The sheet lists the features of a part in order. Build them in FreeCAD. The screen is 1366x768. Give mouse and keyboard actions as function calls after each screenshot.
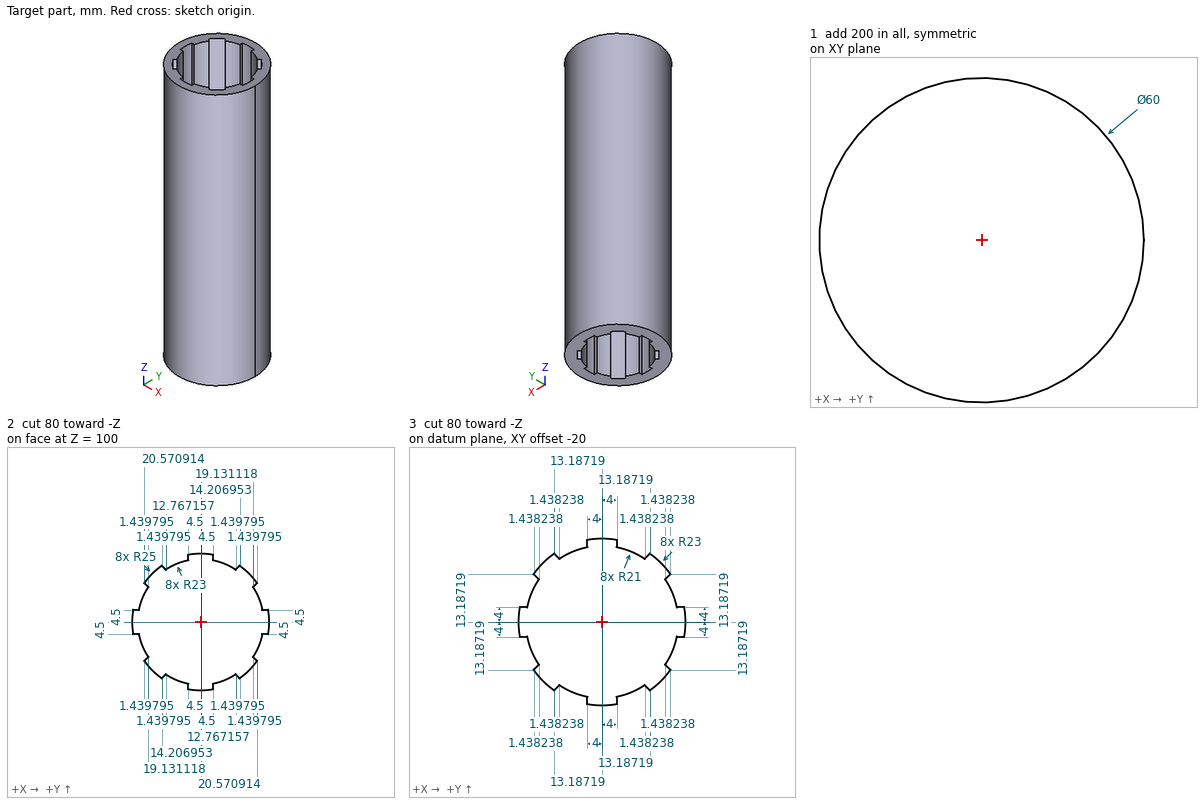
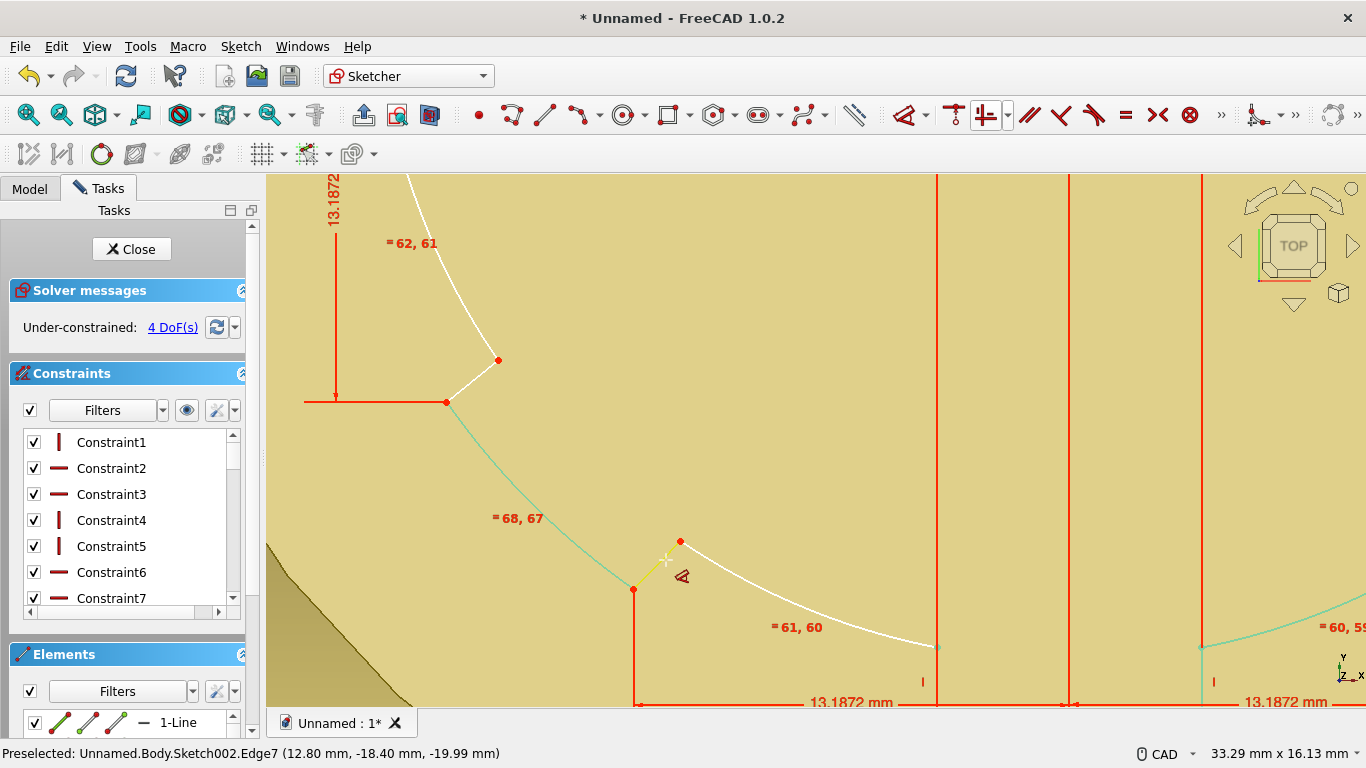
click(667, 556)
click(657, 623)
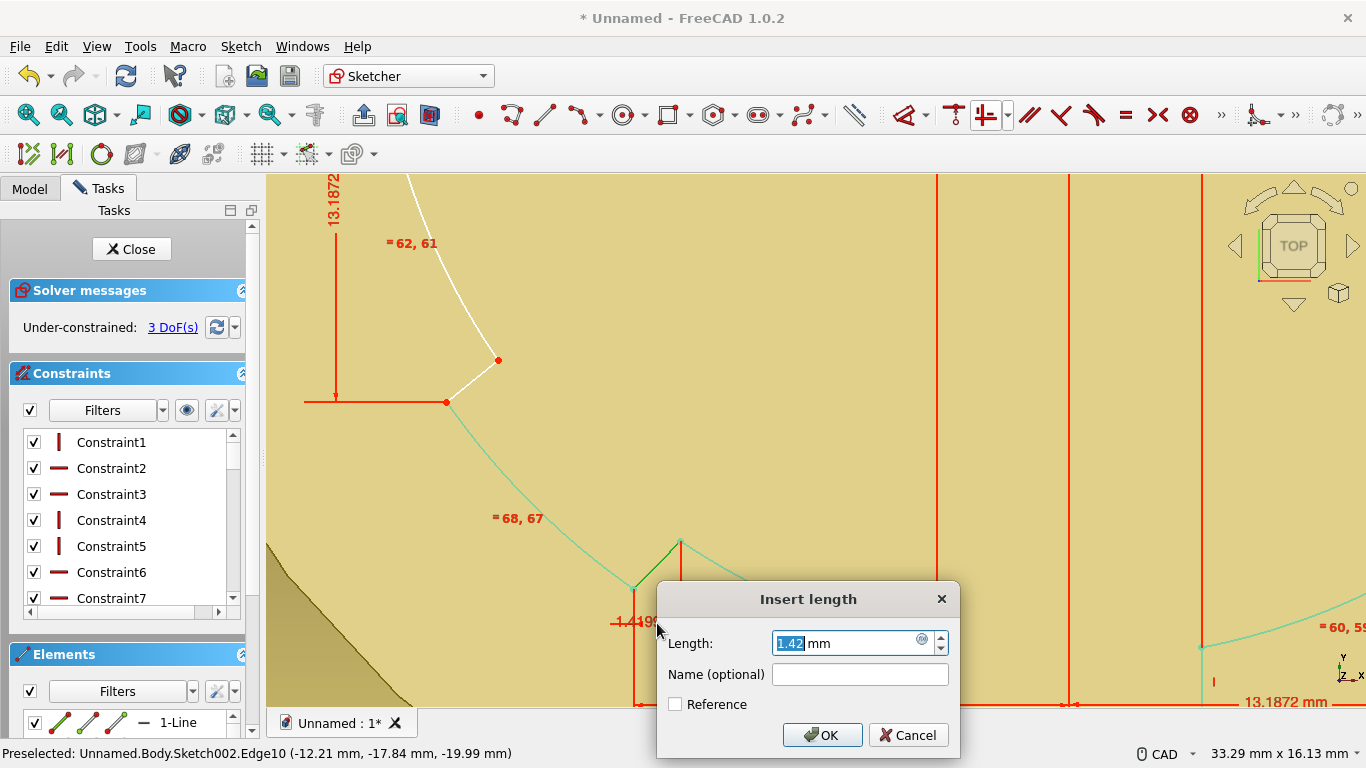
text(1.438238)
key(Return)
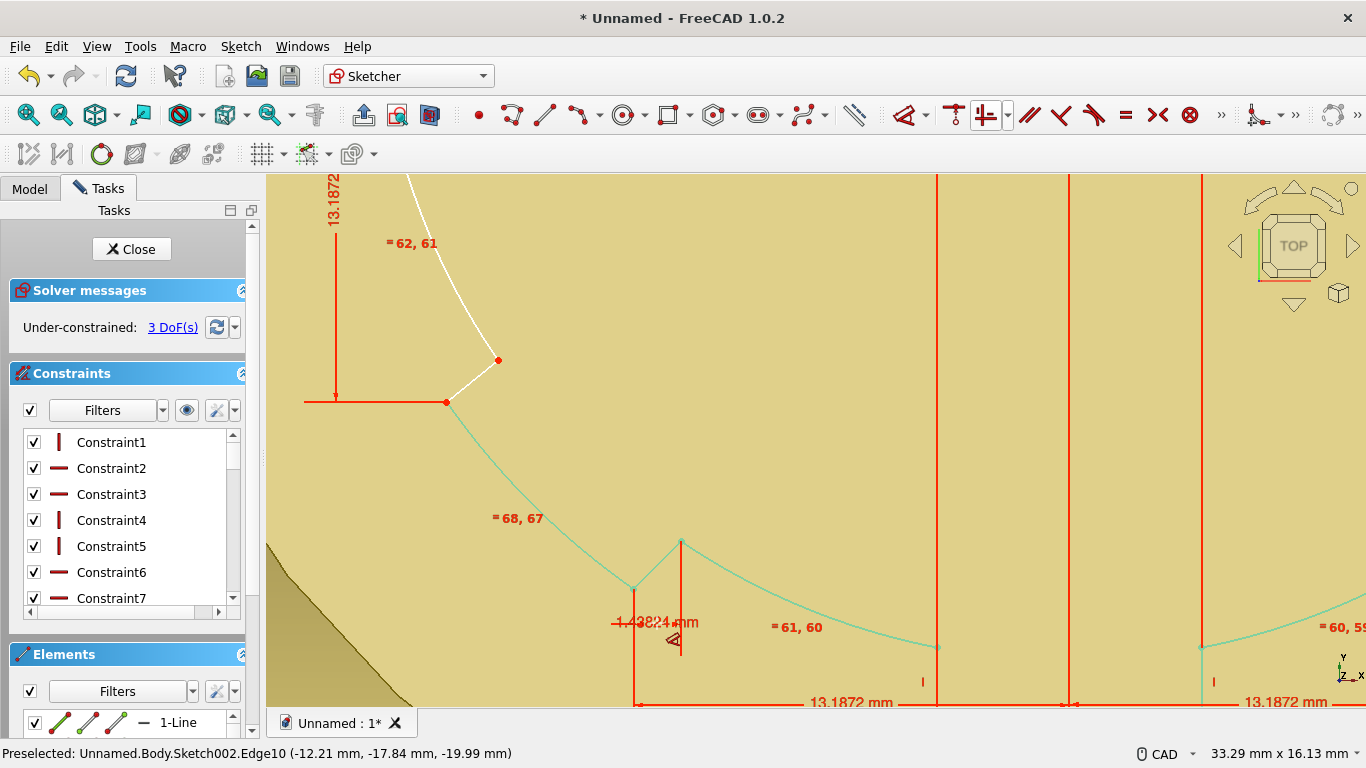
click(462, 390)
click(455, 436)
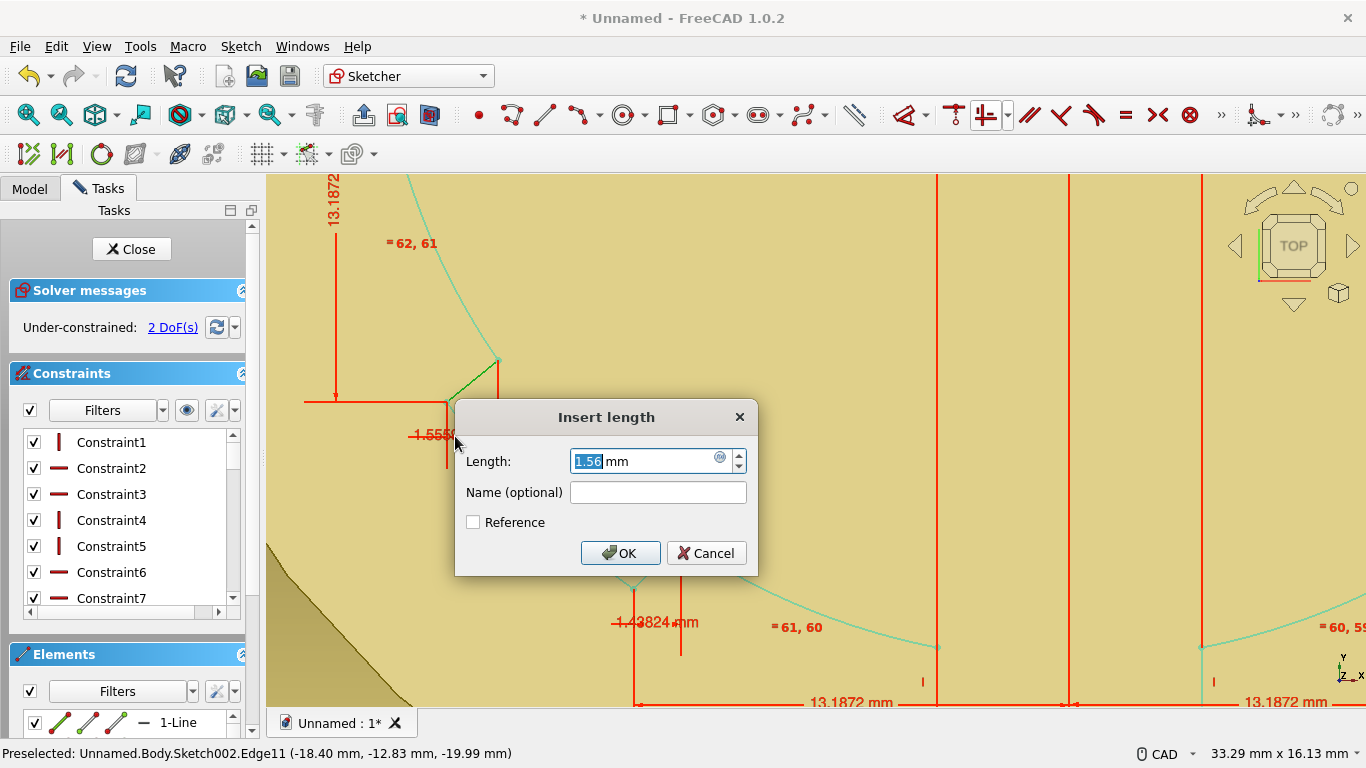
text(1.438238)
key(Return)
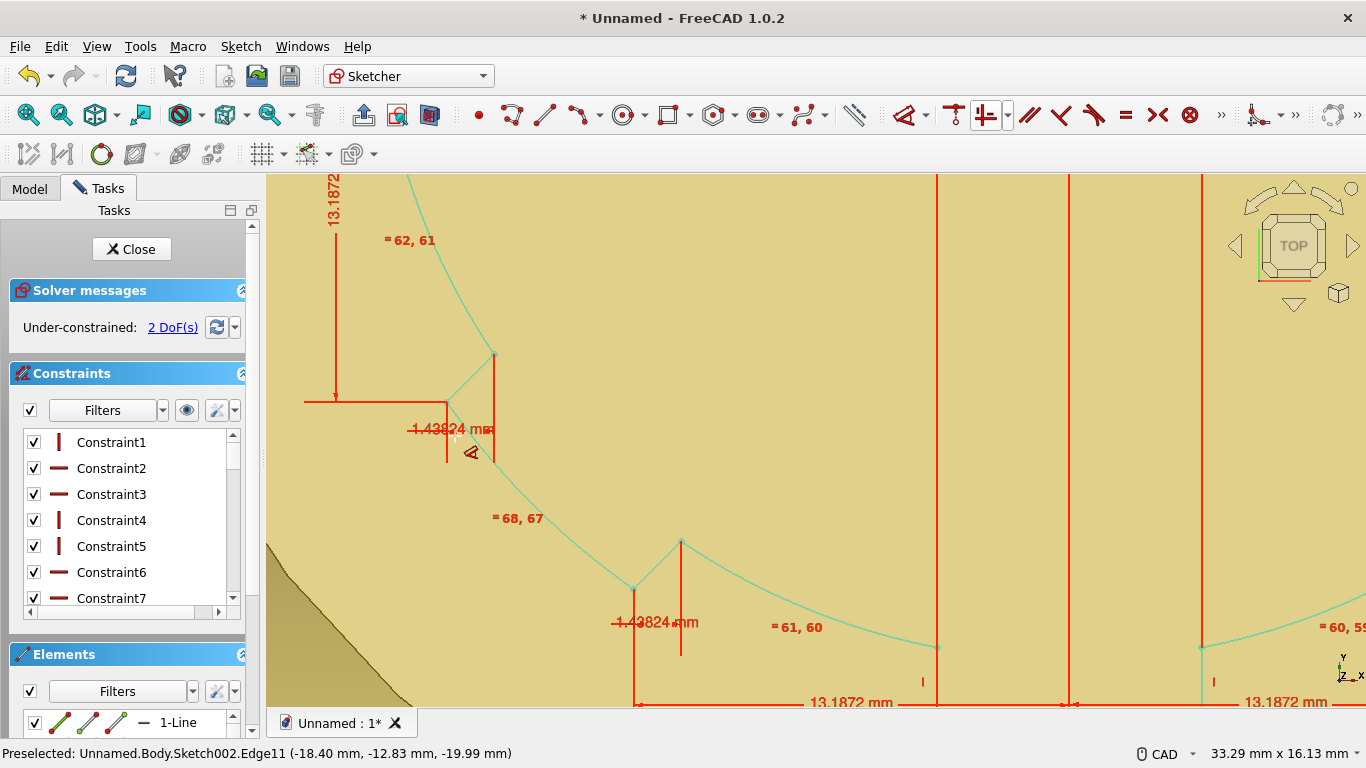
scroll(666, 560, down, 8)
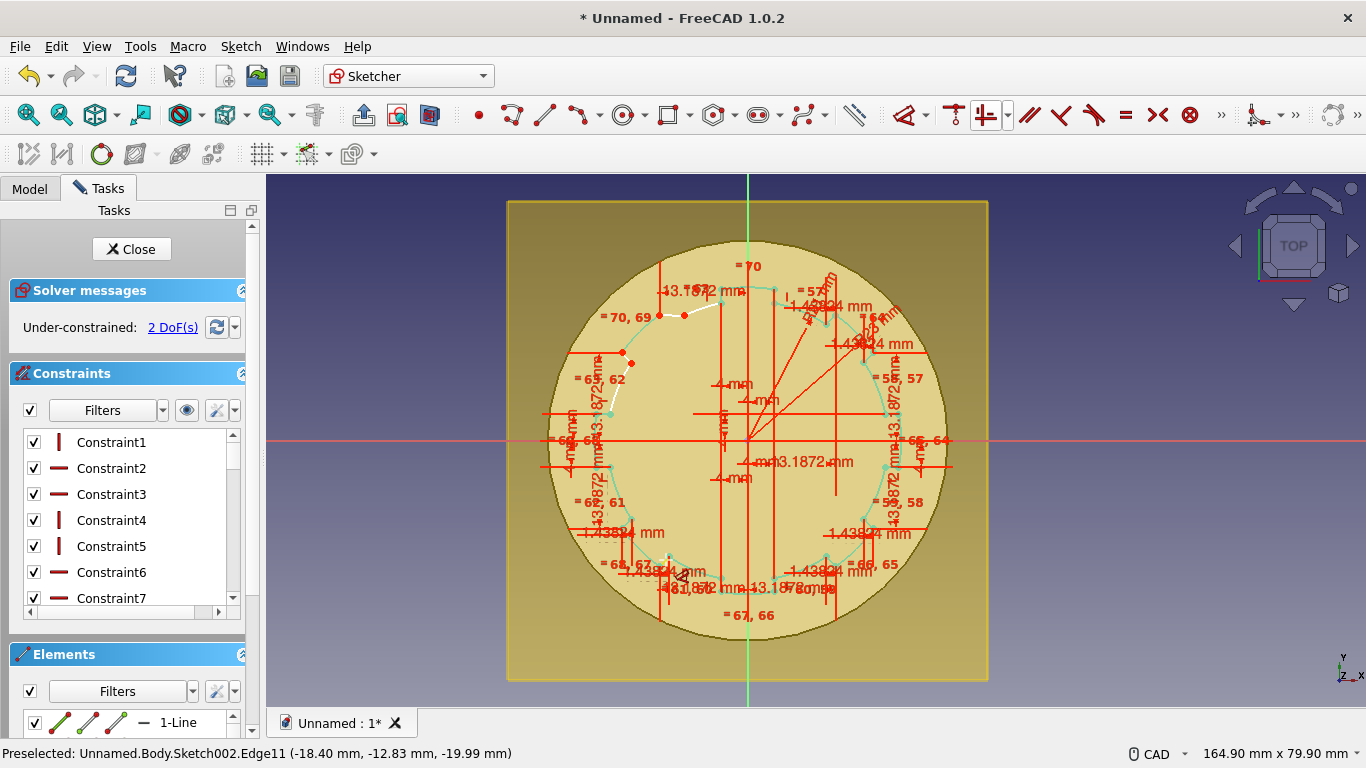
scroll(628, 360, up, 8)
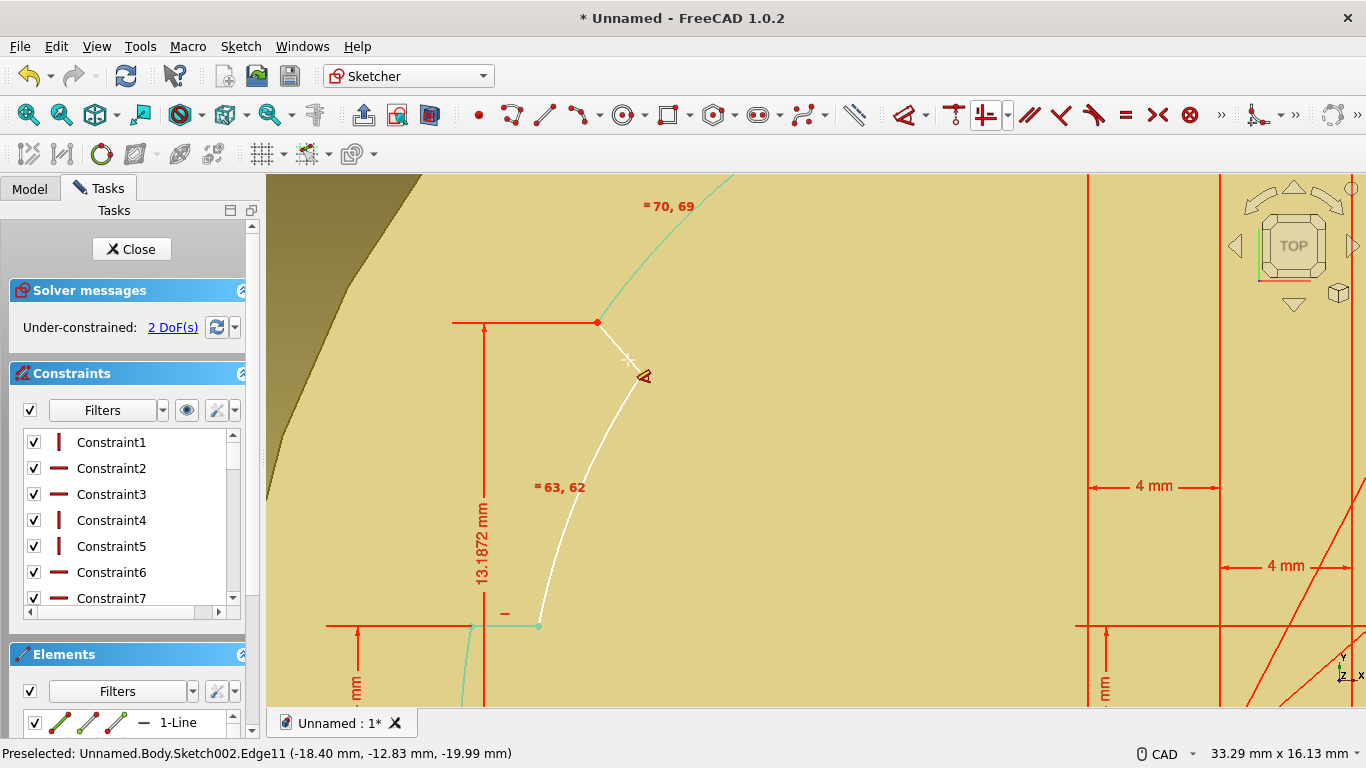
click(629, 359)
click(604, 289)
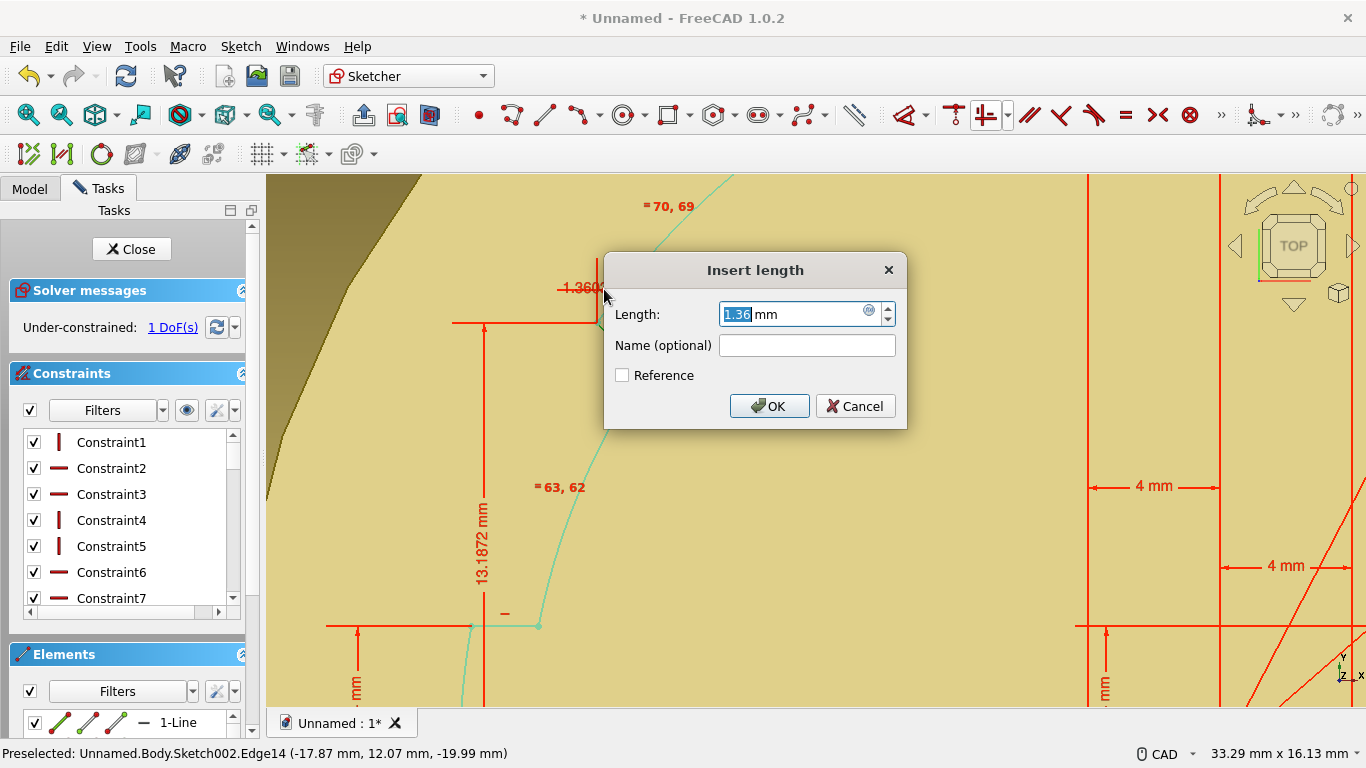
text(1.438238)
key(Return)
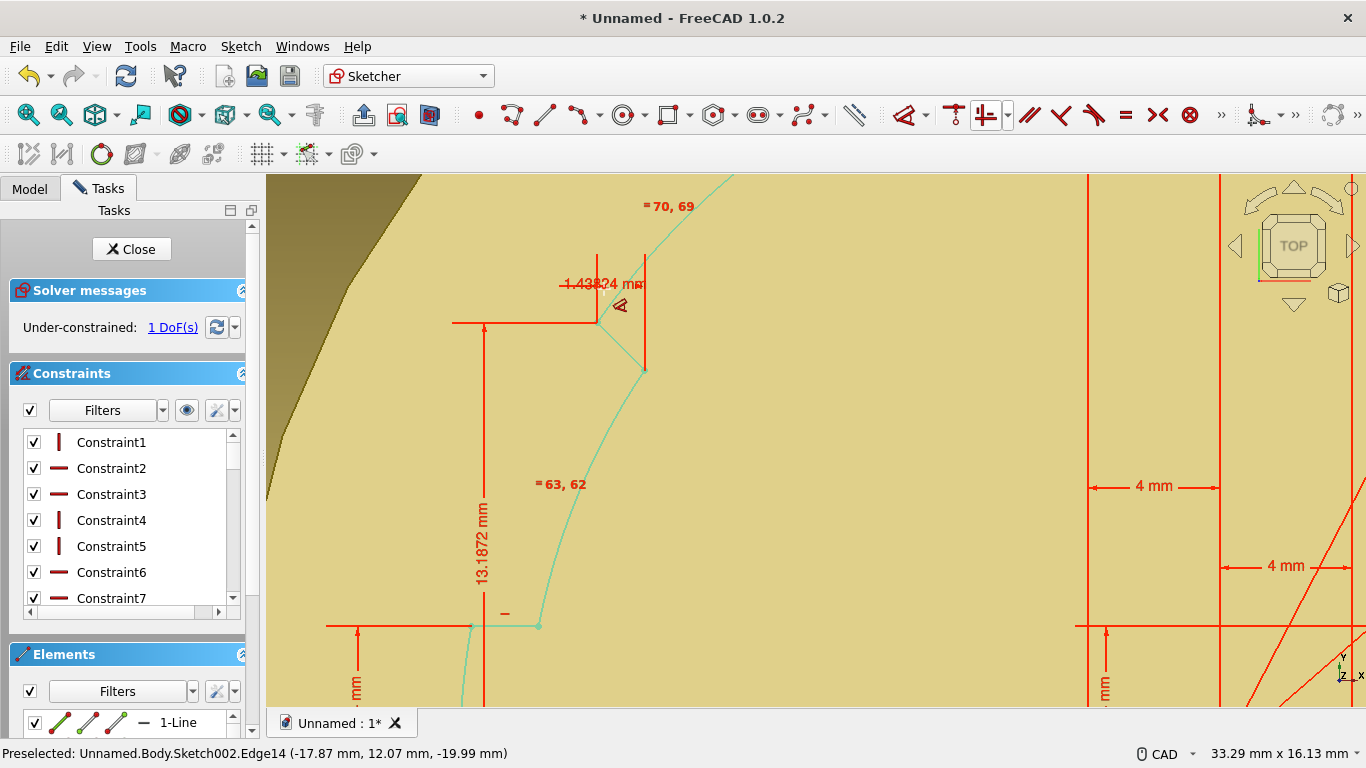
scroll(628, 360, down, 8)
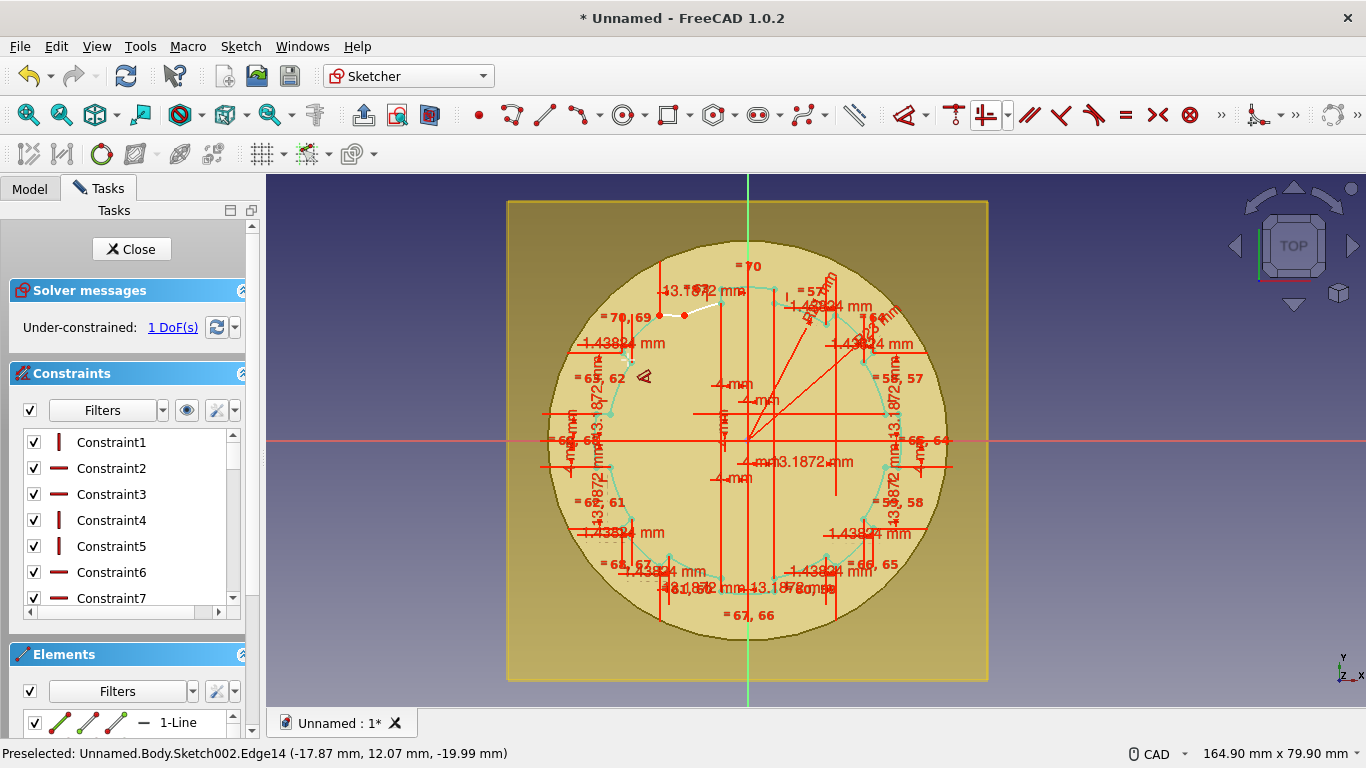
scroll(667, 315, up, 8)